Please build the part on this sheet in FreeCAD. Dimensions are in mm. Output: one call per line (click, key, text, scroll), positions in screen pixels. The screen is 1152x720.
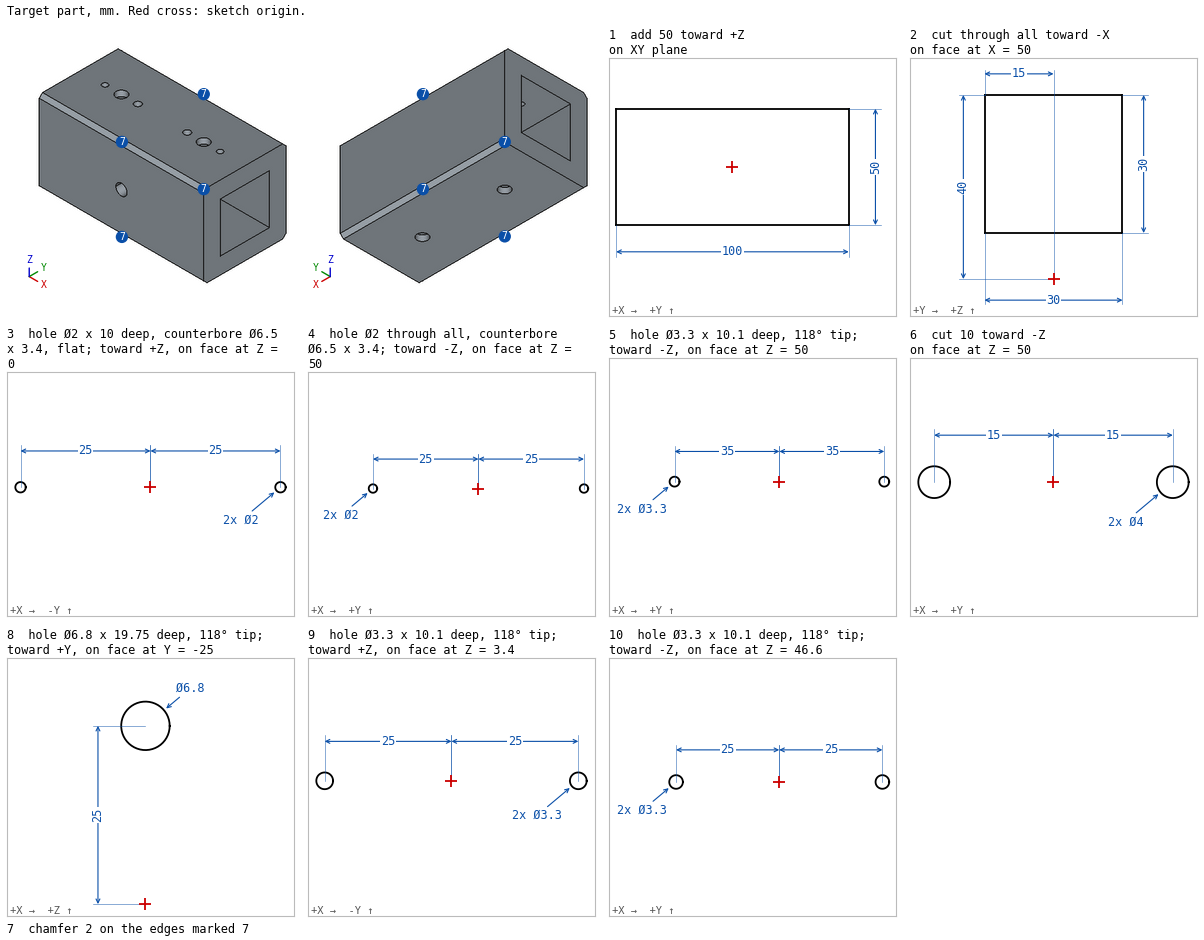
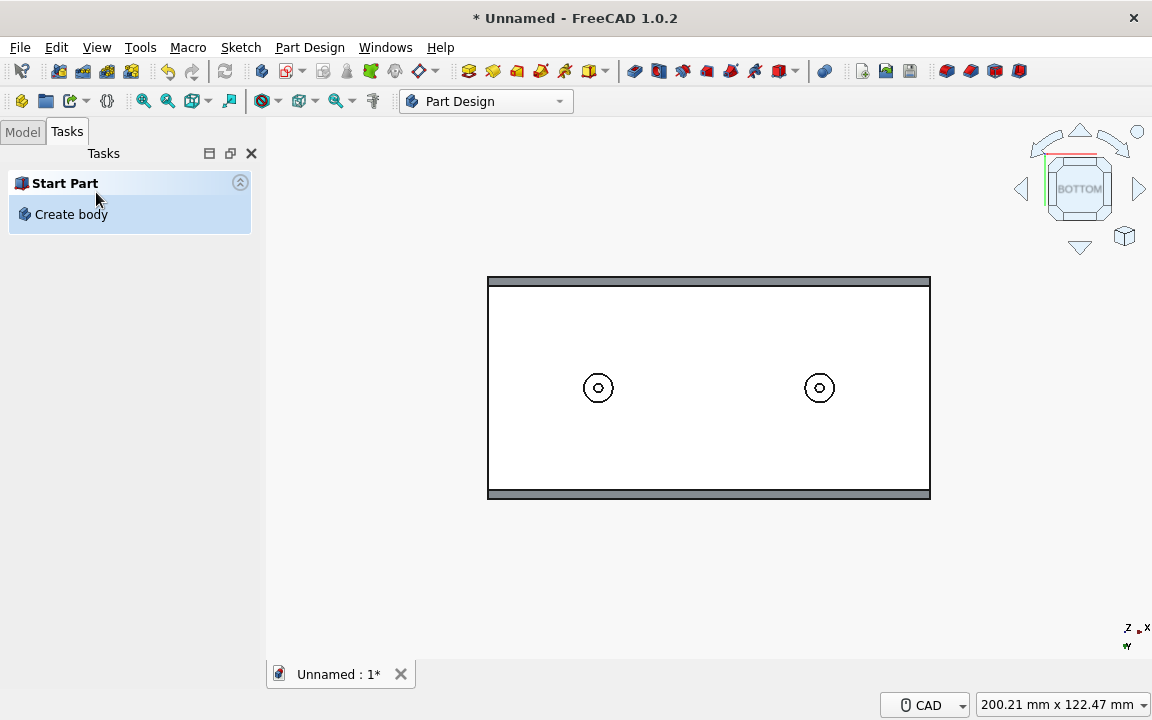
key(0)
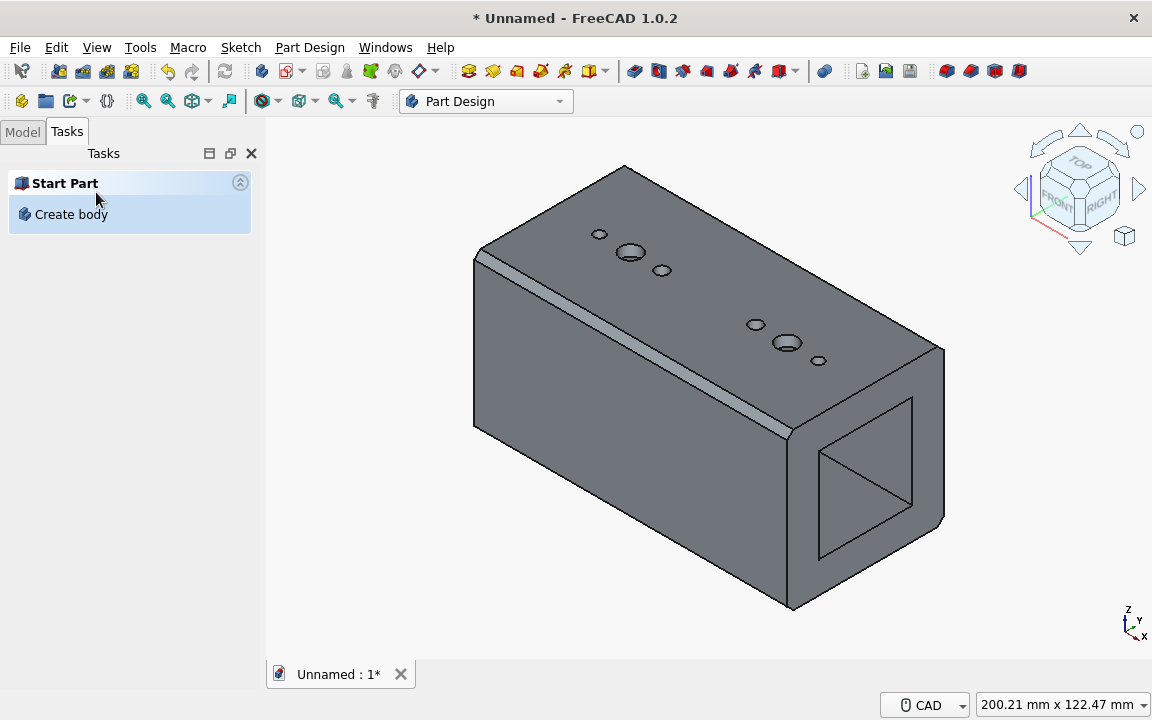
click(675, 458)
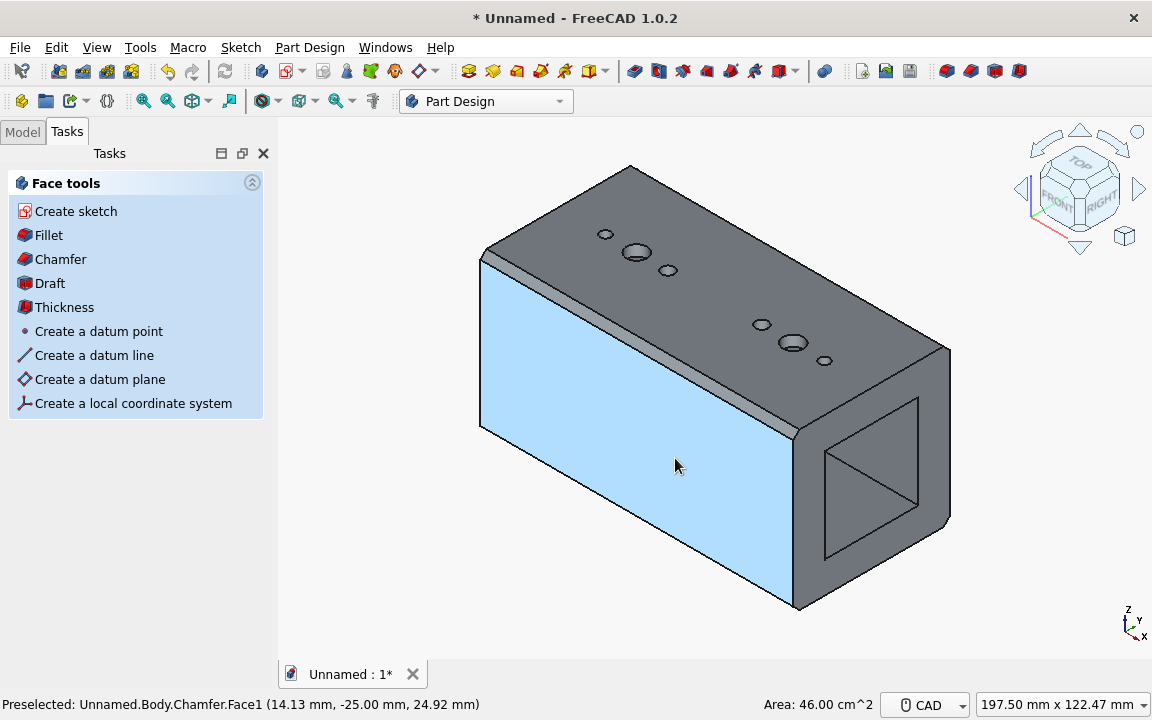
click(286, 72)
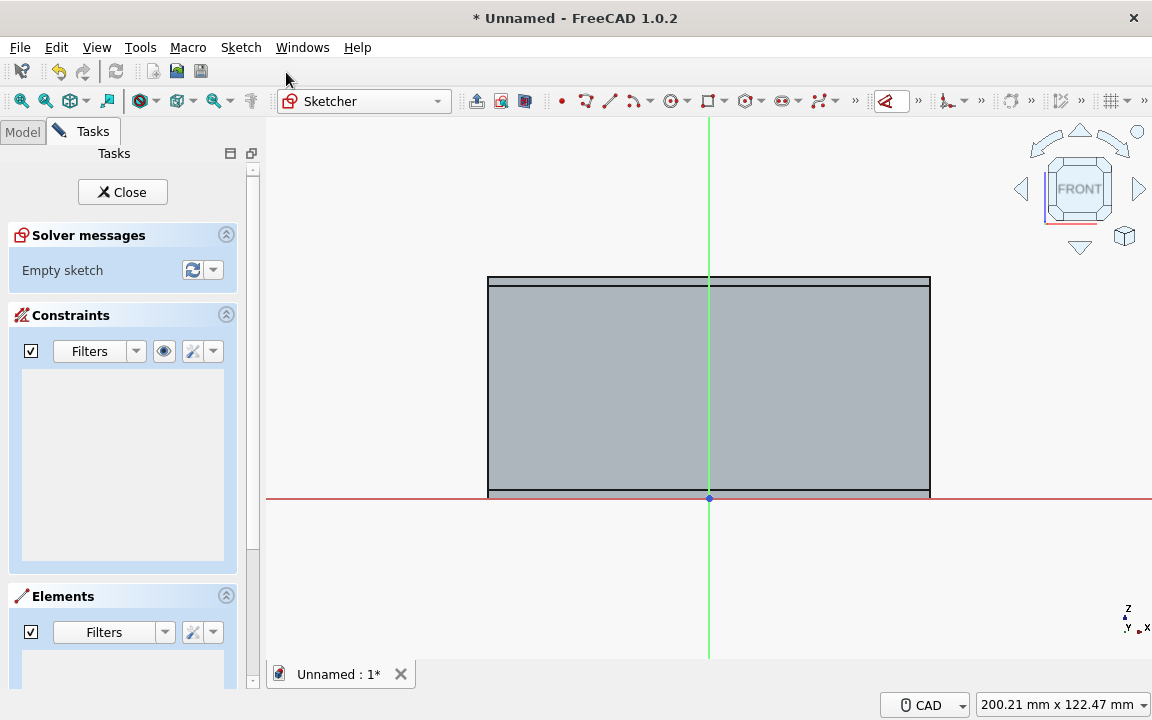
scroll(716, 388, up, 12)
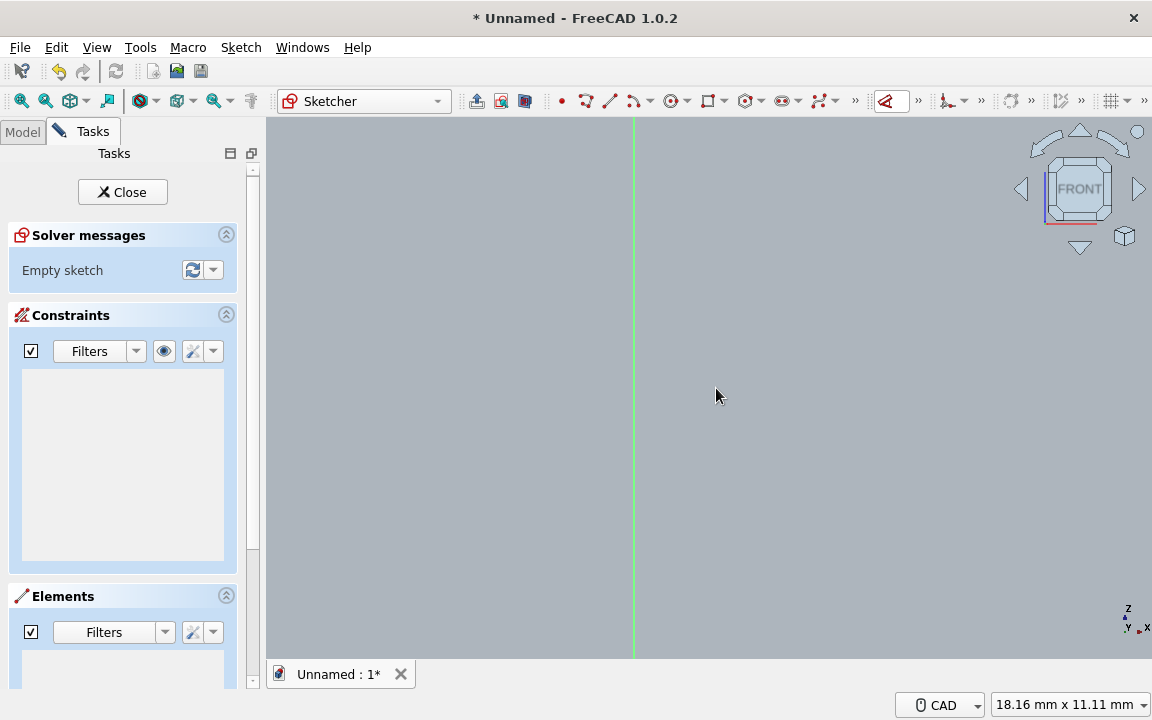
click(672, 102)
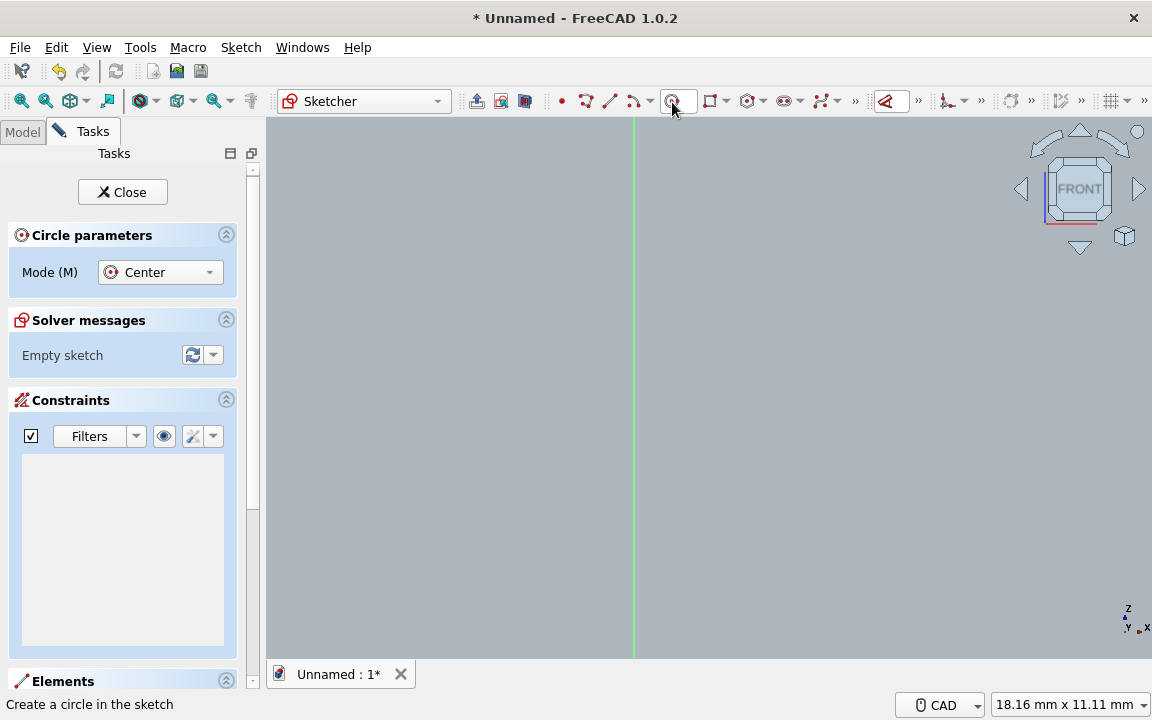
click(634, 383)
move(751, 266)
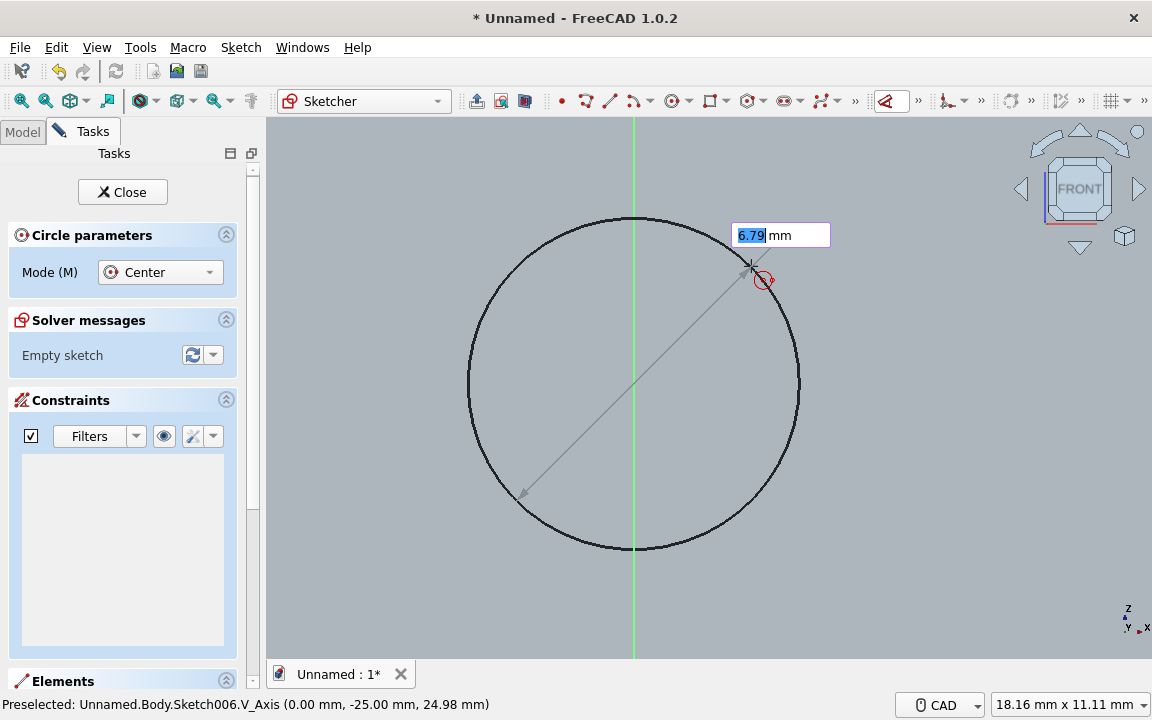
text(6.8)
key(Return)
key(Escape)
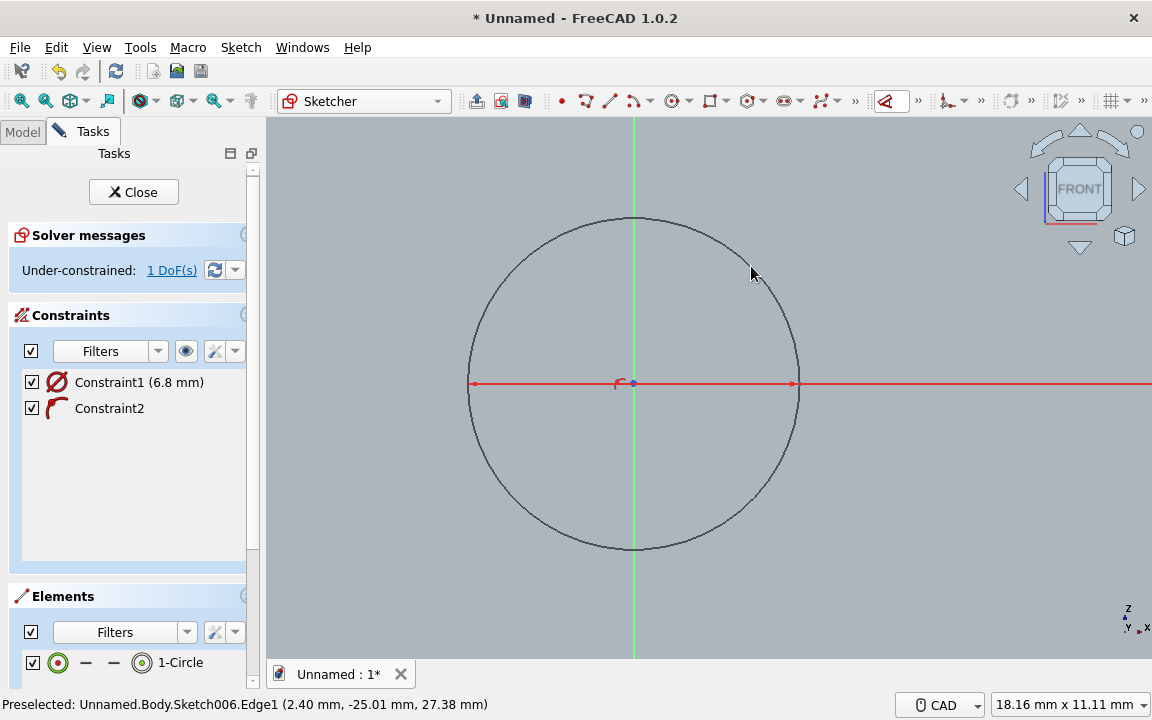
click(634, 384)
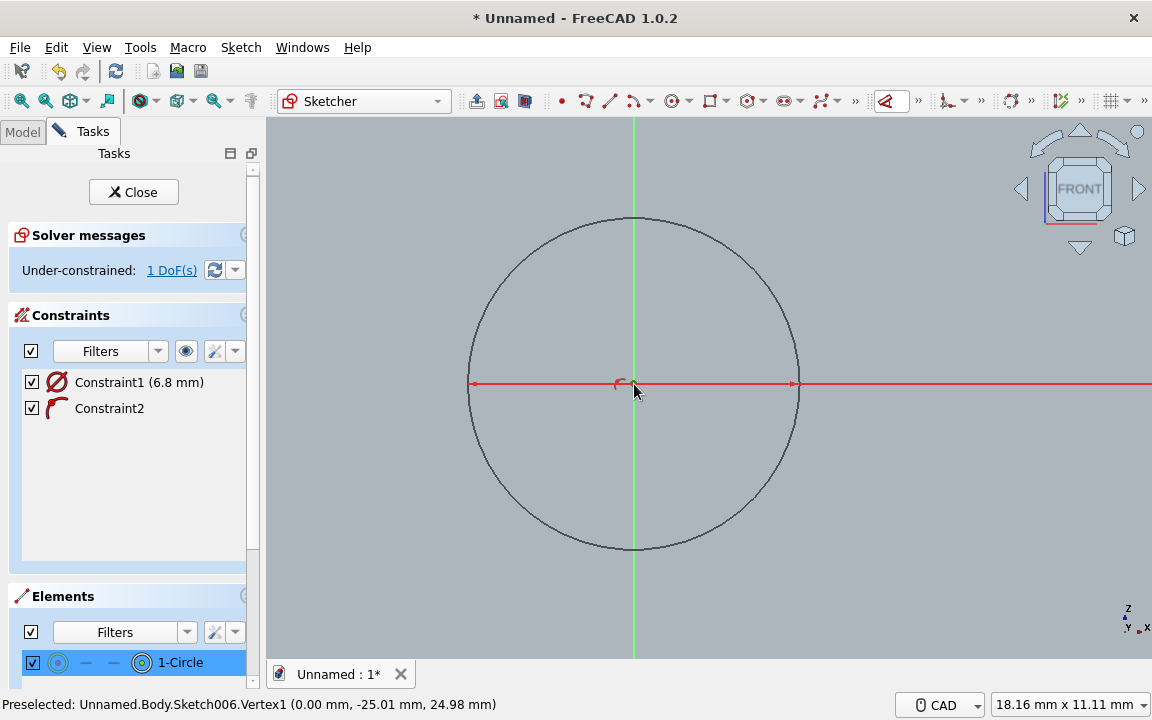
key(i)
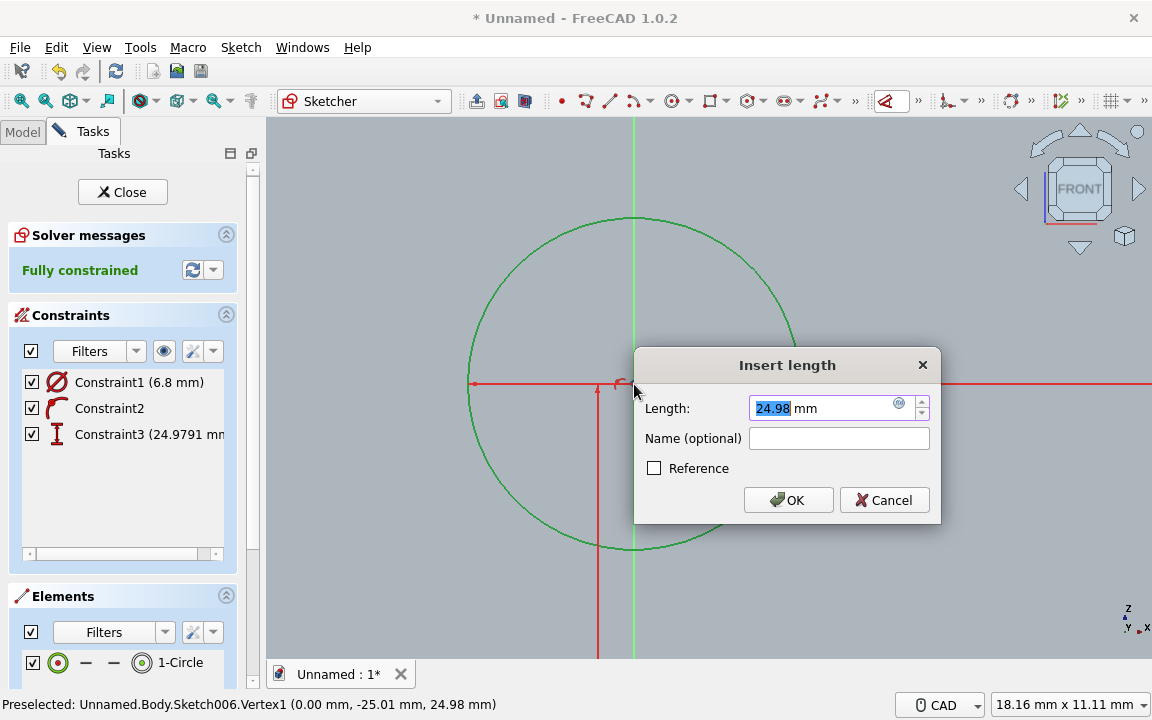
text(25)
key(Return)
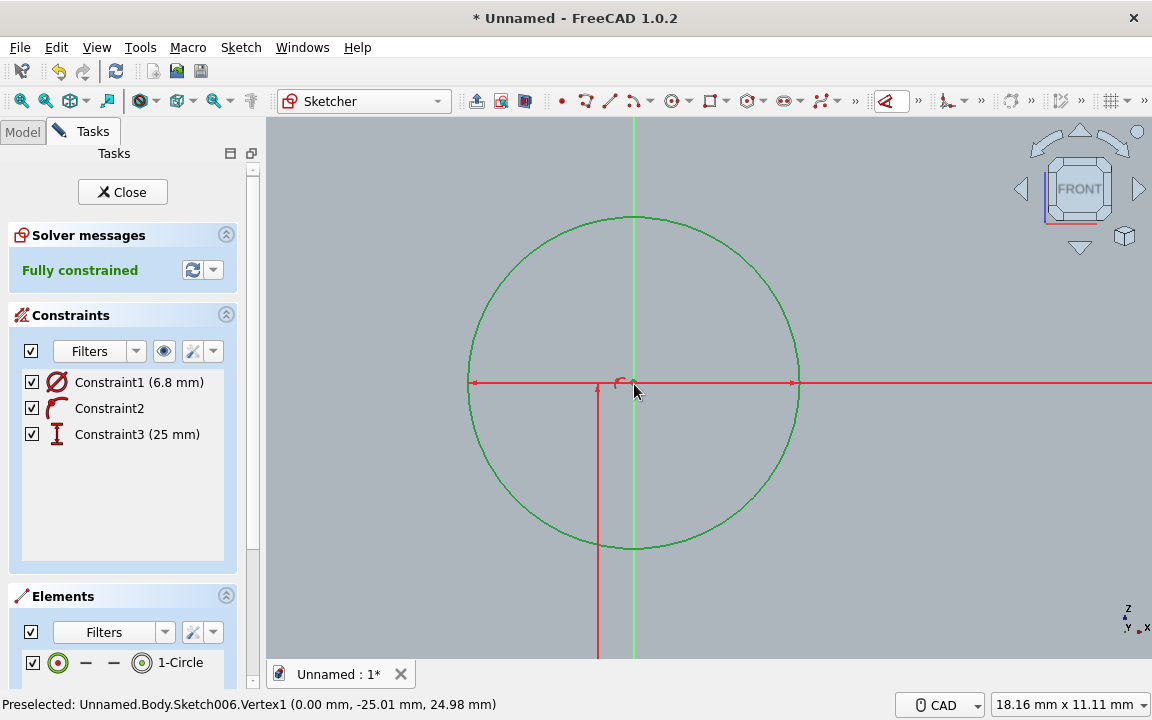
click(123, 192)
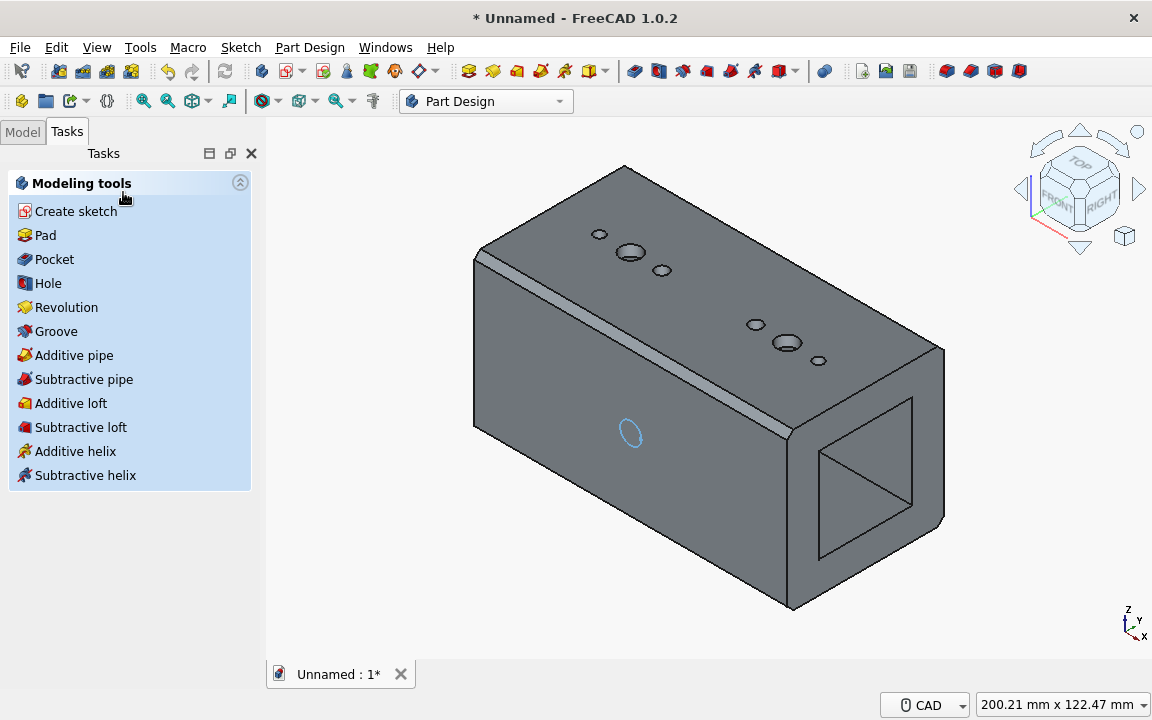
click(660, 72)